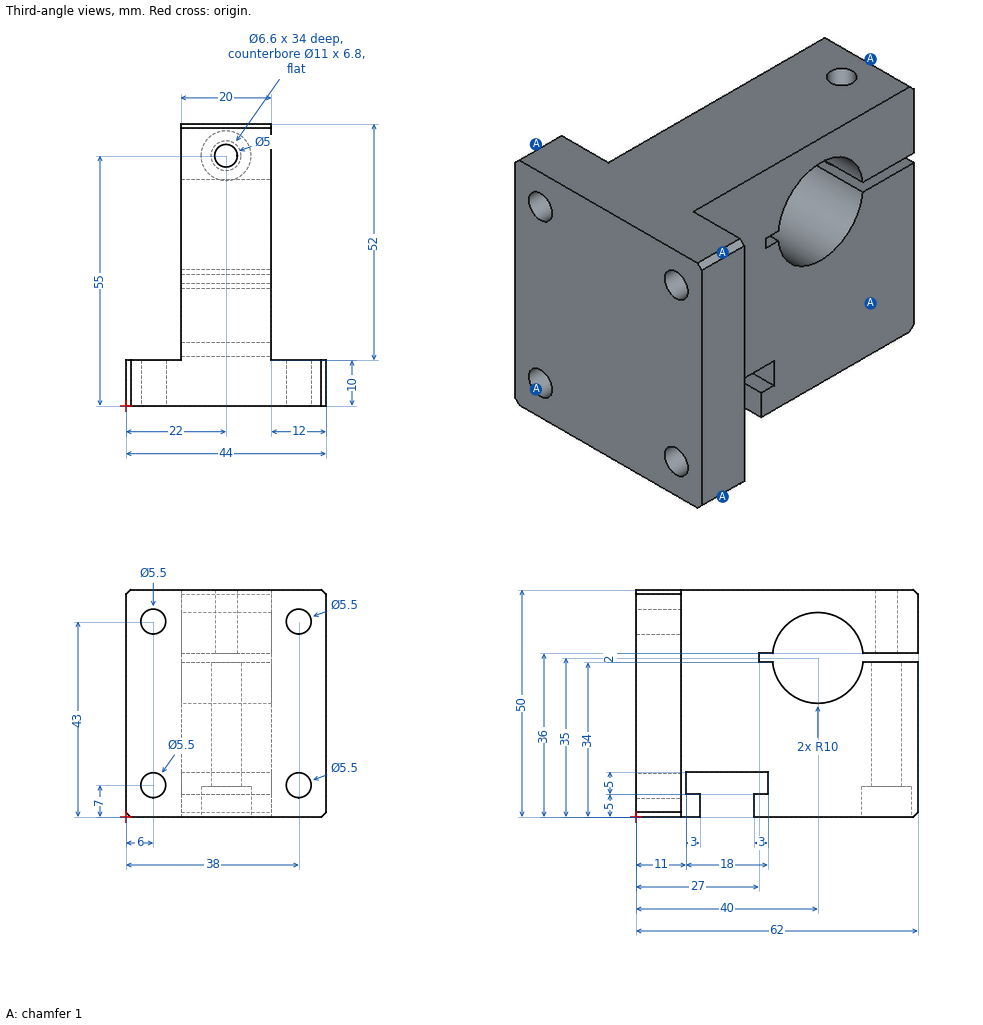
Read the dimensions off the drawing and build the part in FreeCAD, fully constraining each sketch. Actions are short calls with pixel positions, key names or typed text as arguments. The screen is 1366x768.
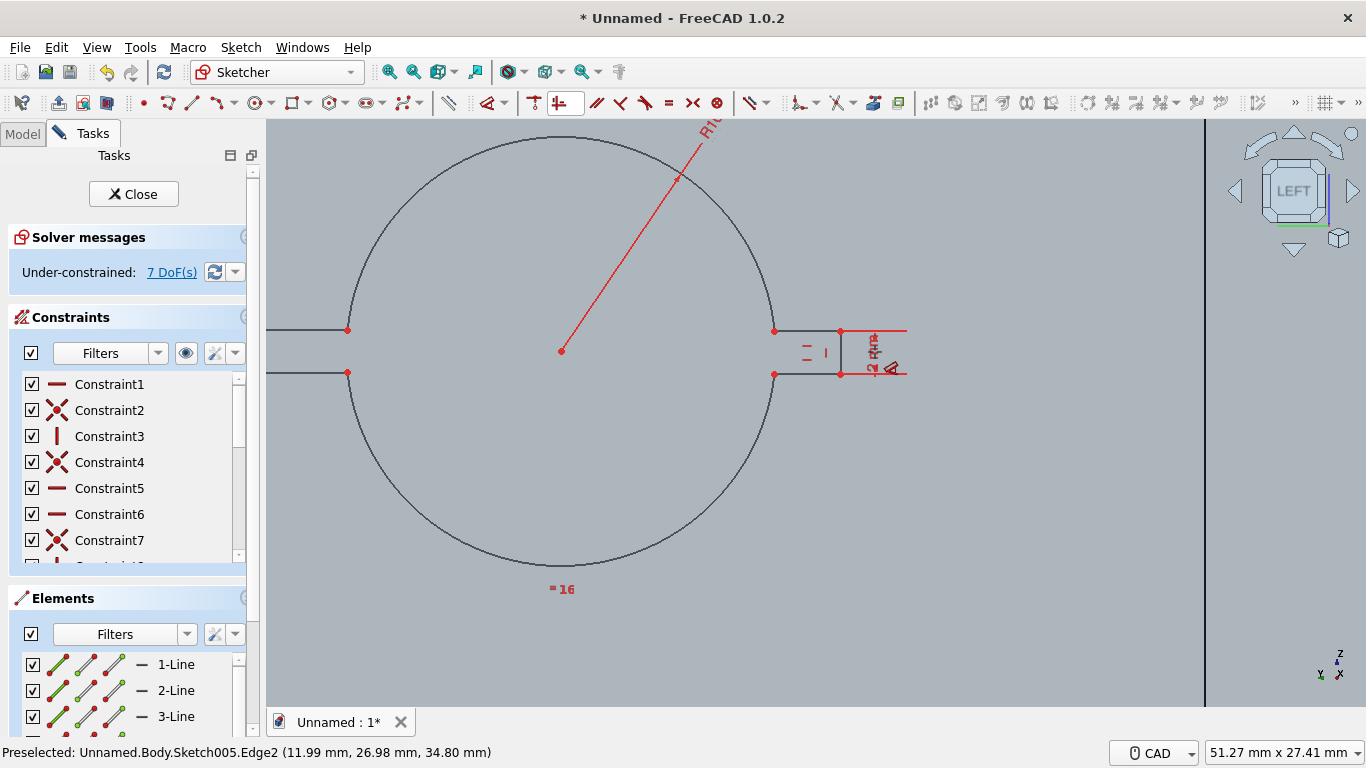
scroll(743, 294, down, 5)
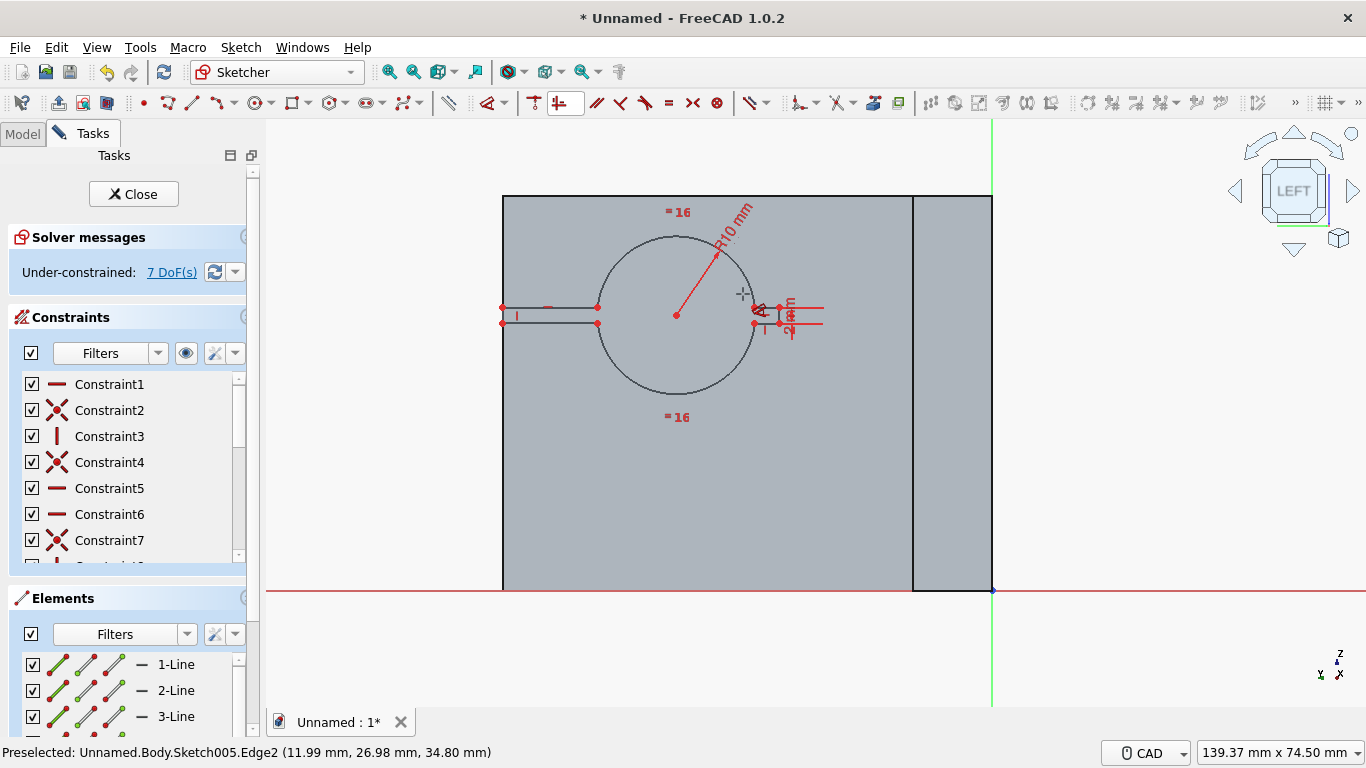
scroll(503, 312, up, 6)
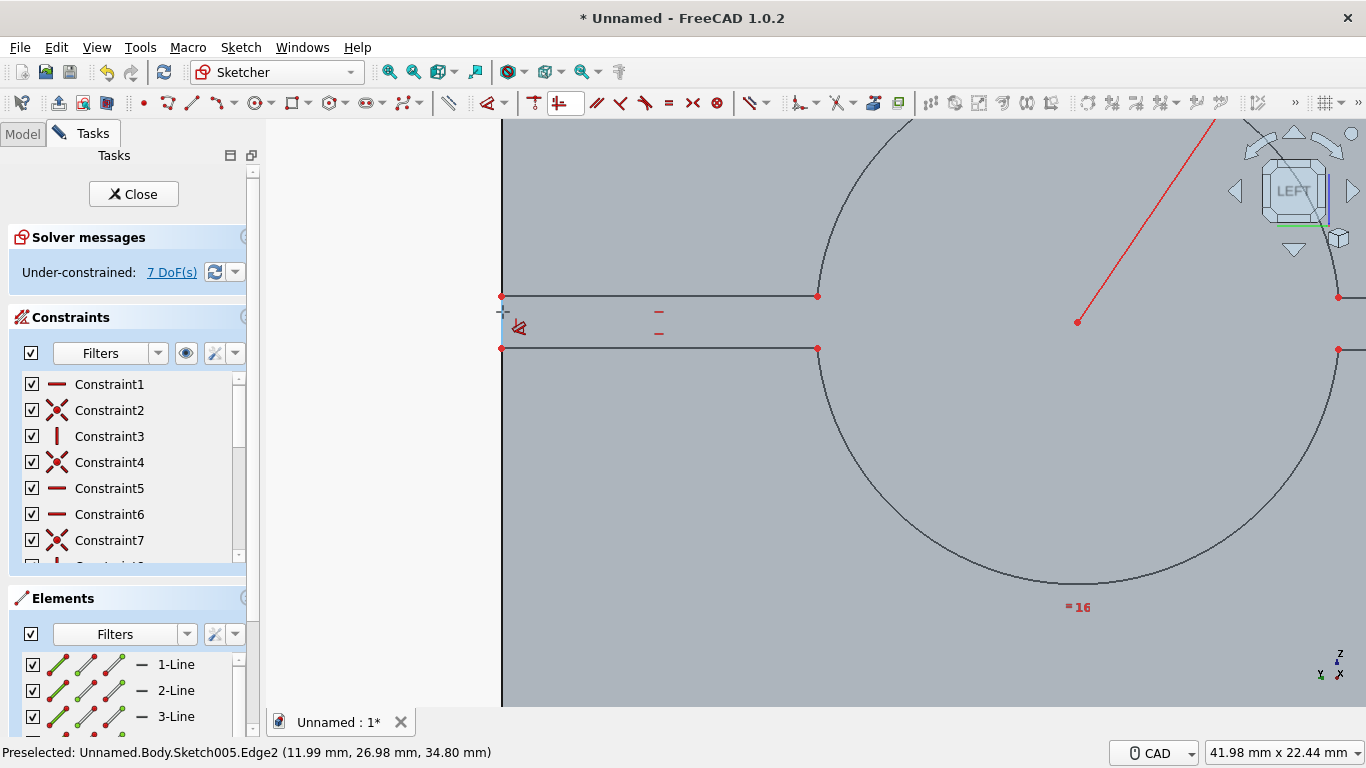
click(502, 312)
click(468, 322)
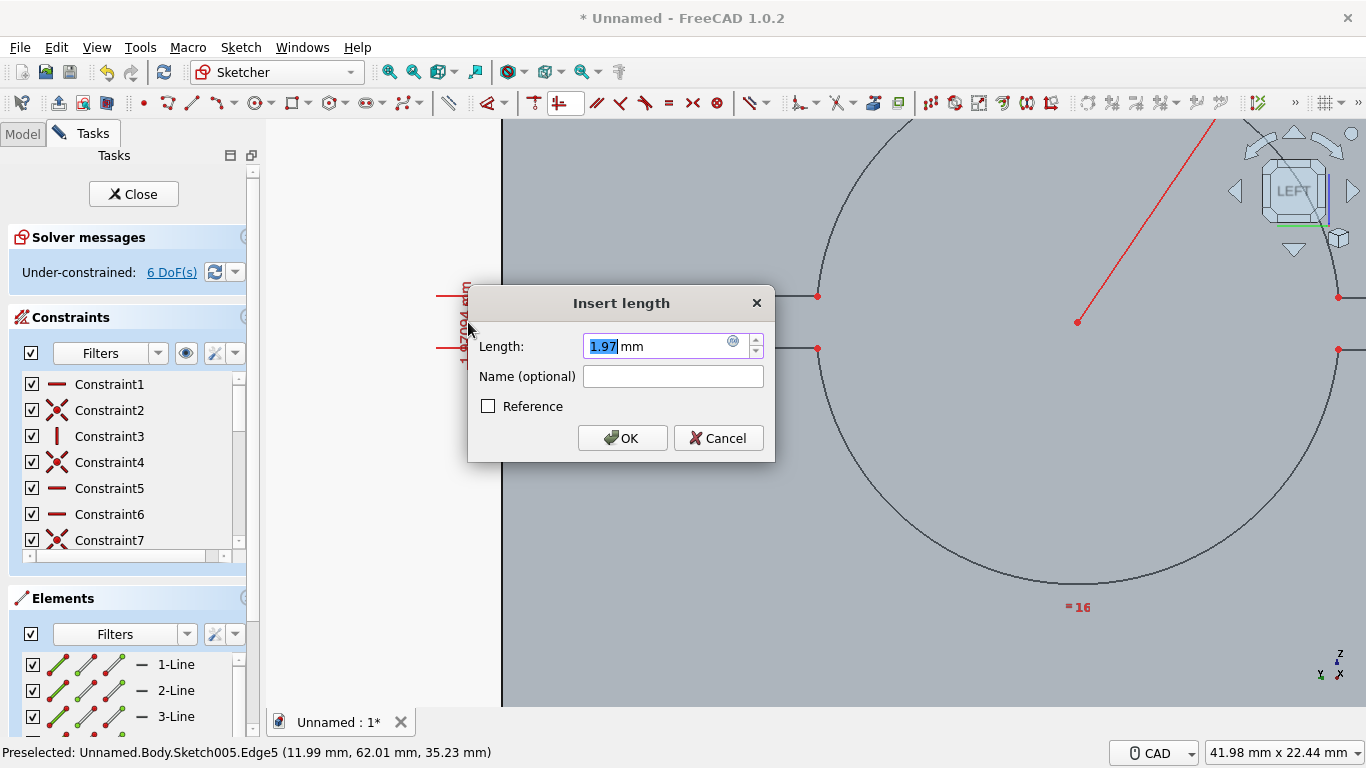
text(2)
key(Return)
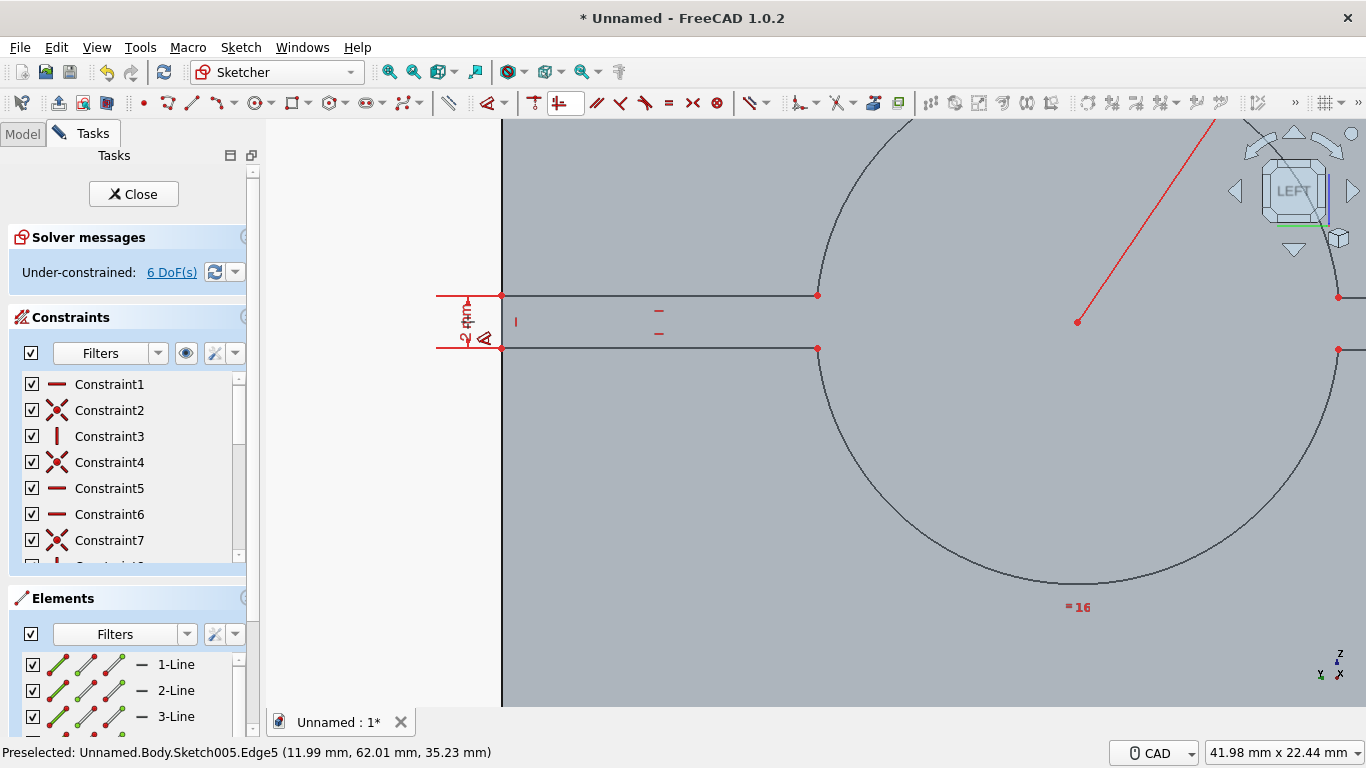
scroll(503, 312, down, 6)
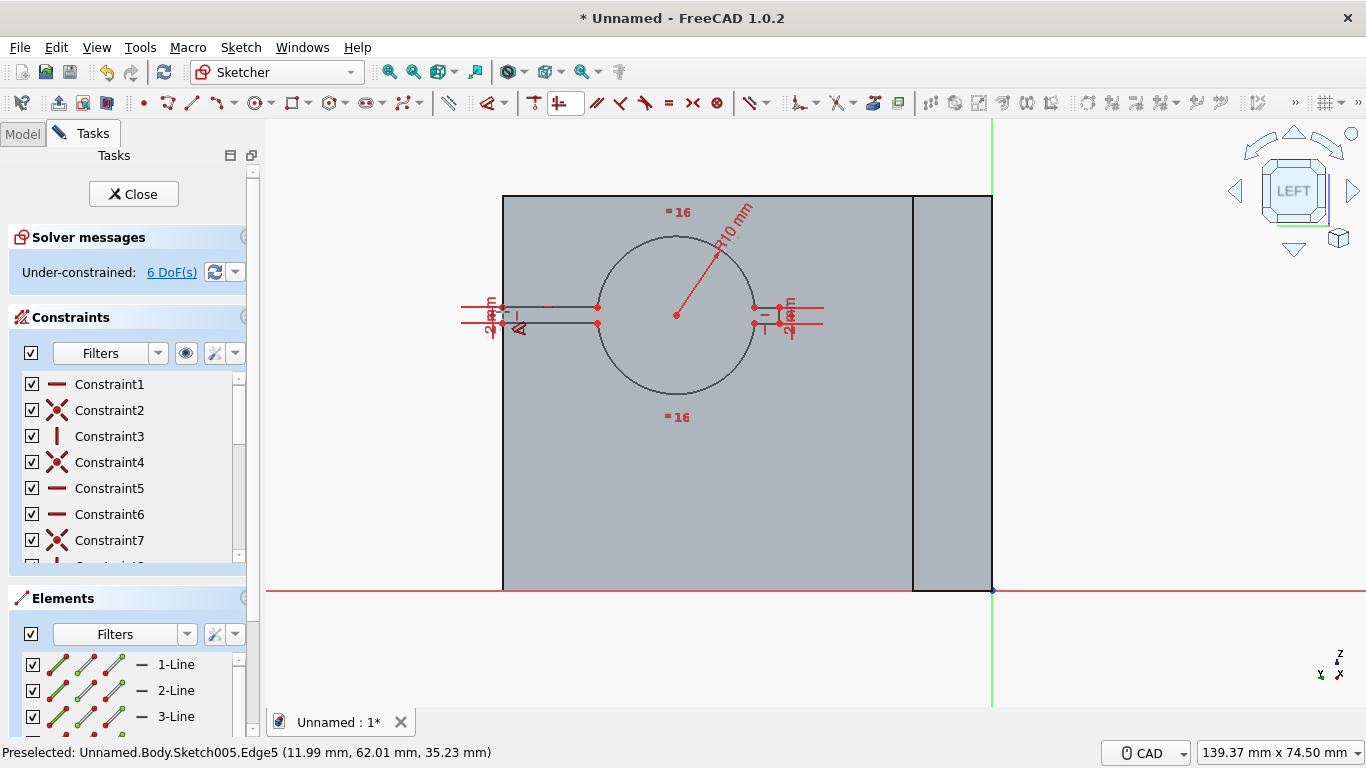
click(755, 324)
click(1026, 457)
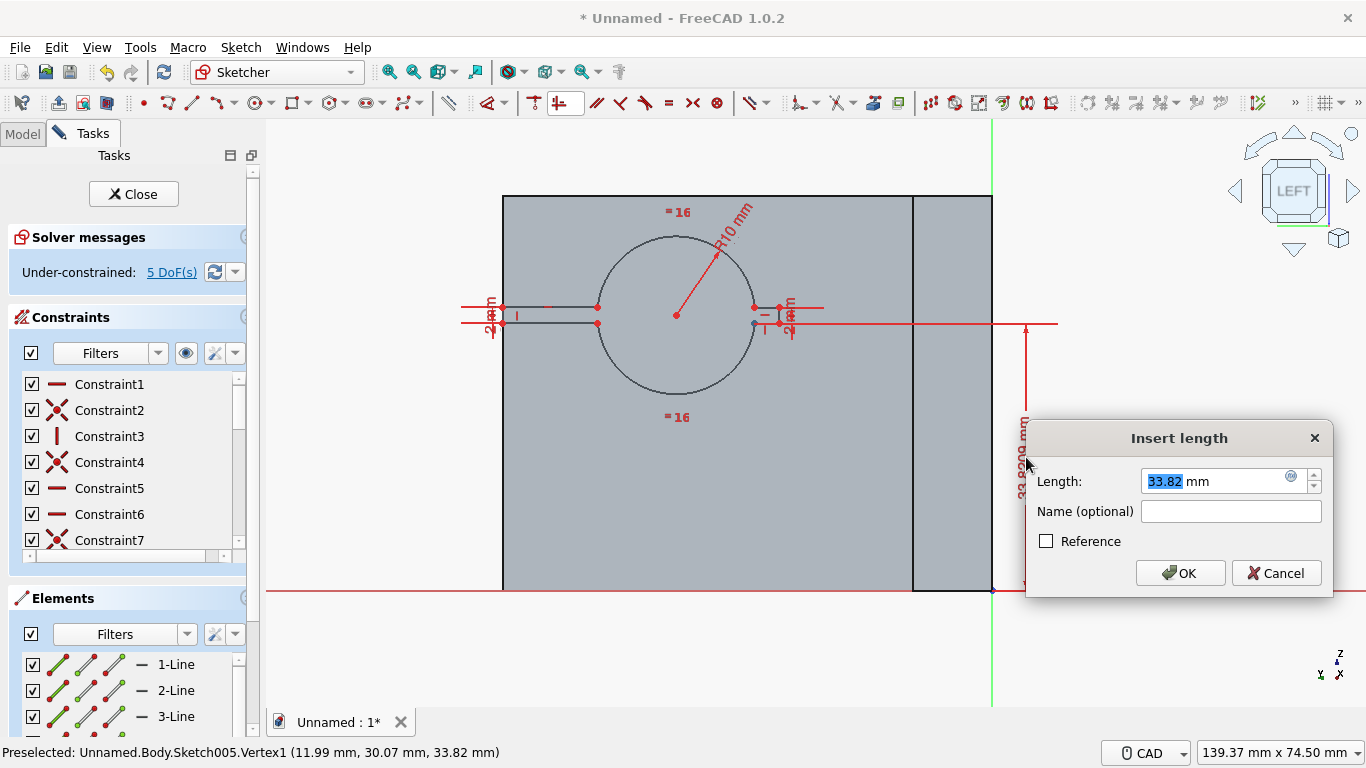
text(34)
key(Return)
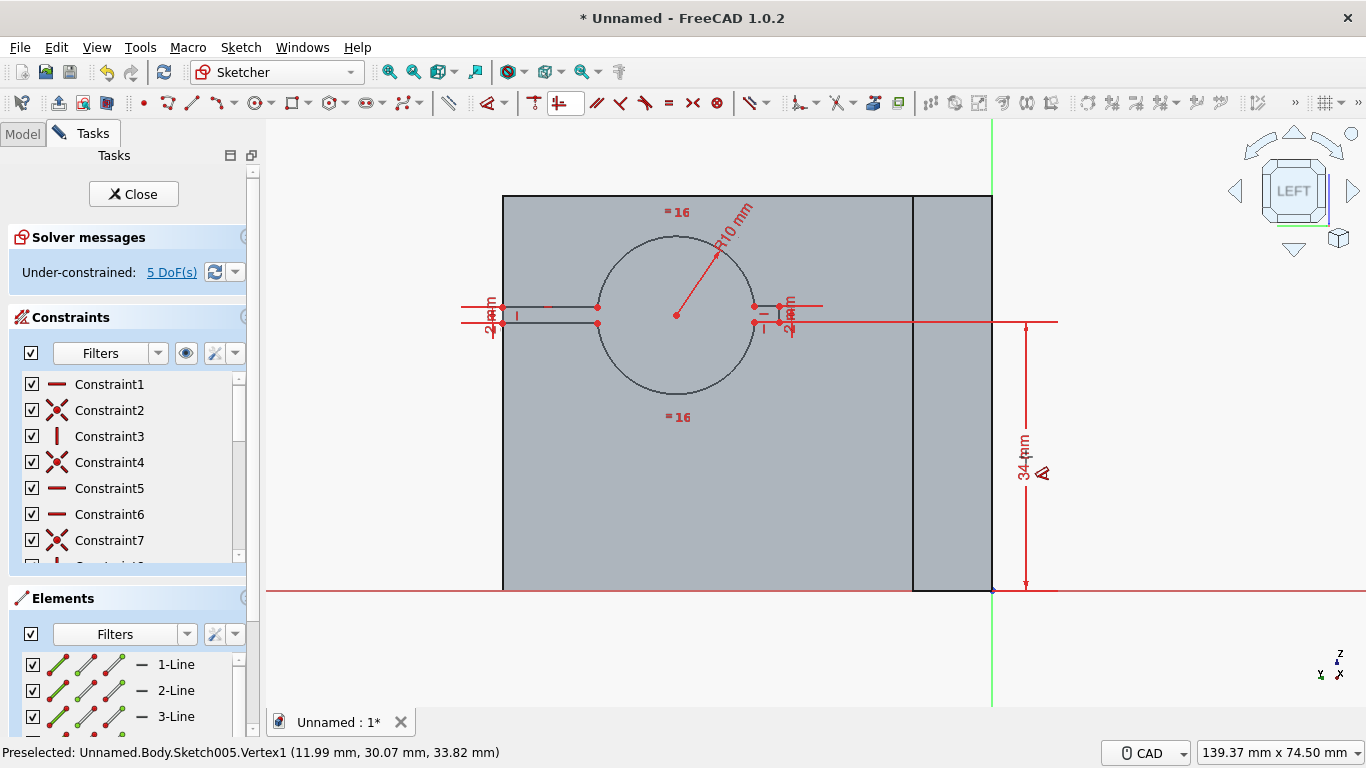
click(779, 322)
click(886, 625)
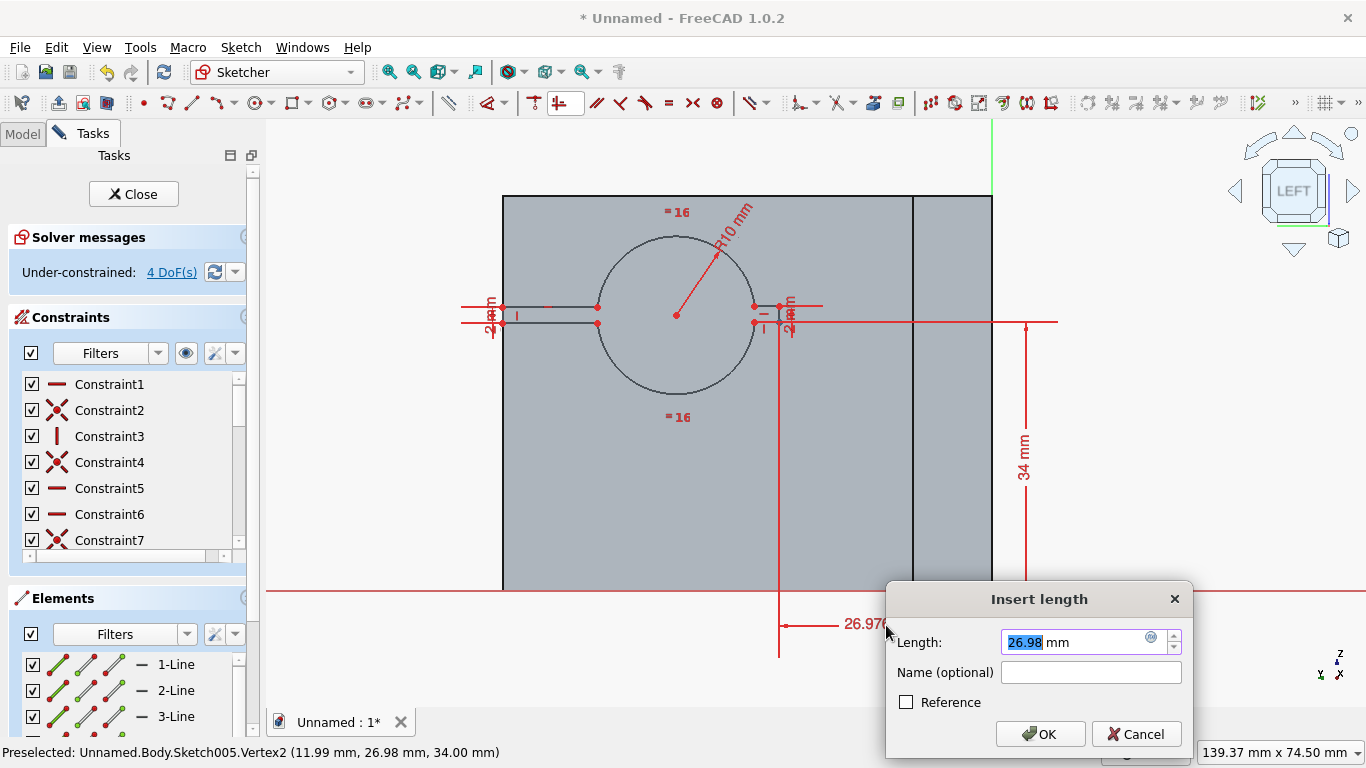
text(27)
key(Return)